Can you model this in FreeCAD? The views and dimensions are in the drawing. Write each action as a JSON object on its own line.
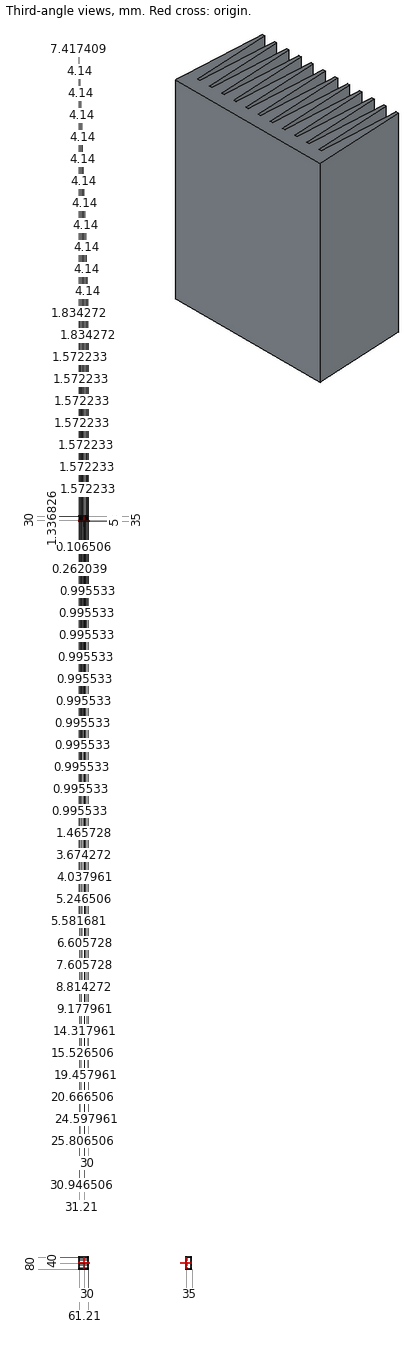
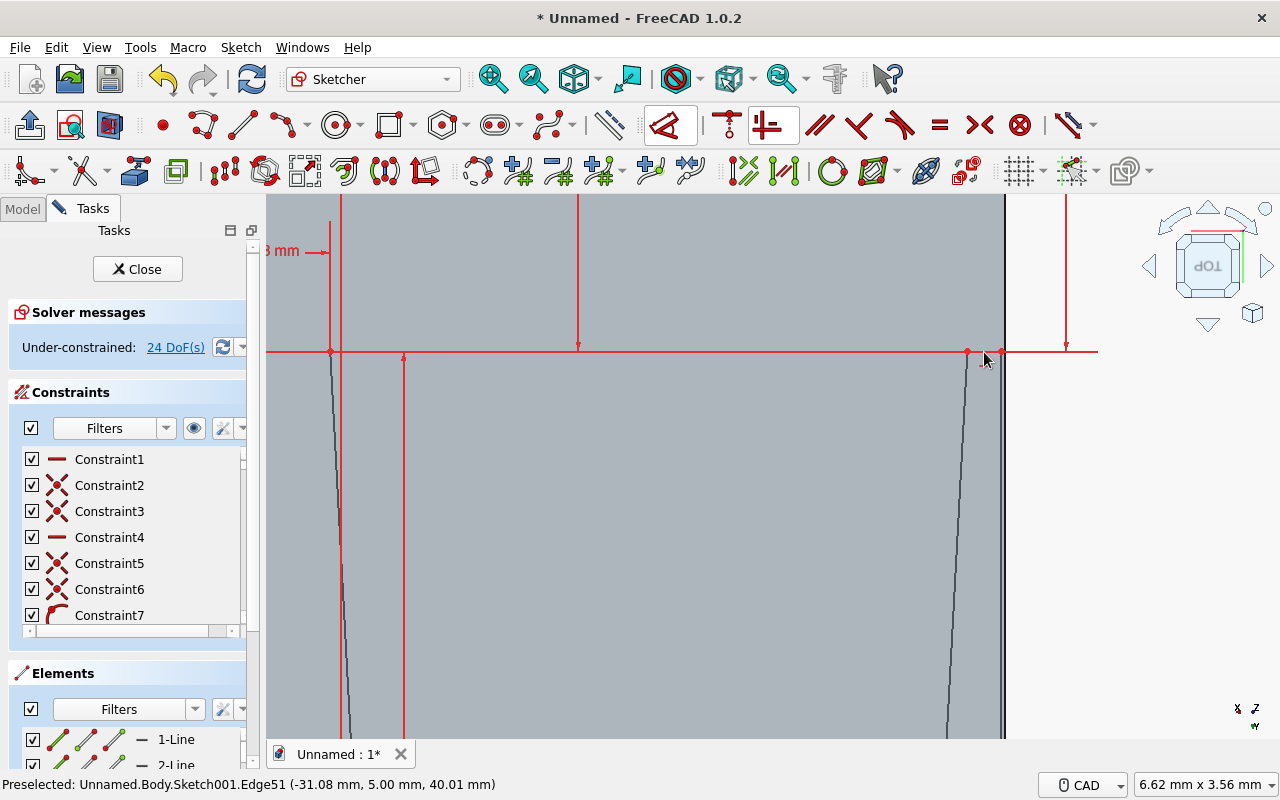
{"action": "left_click", "coordinate": [692, 126]}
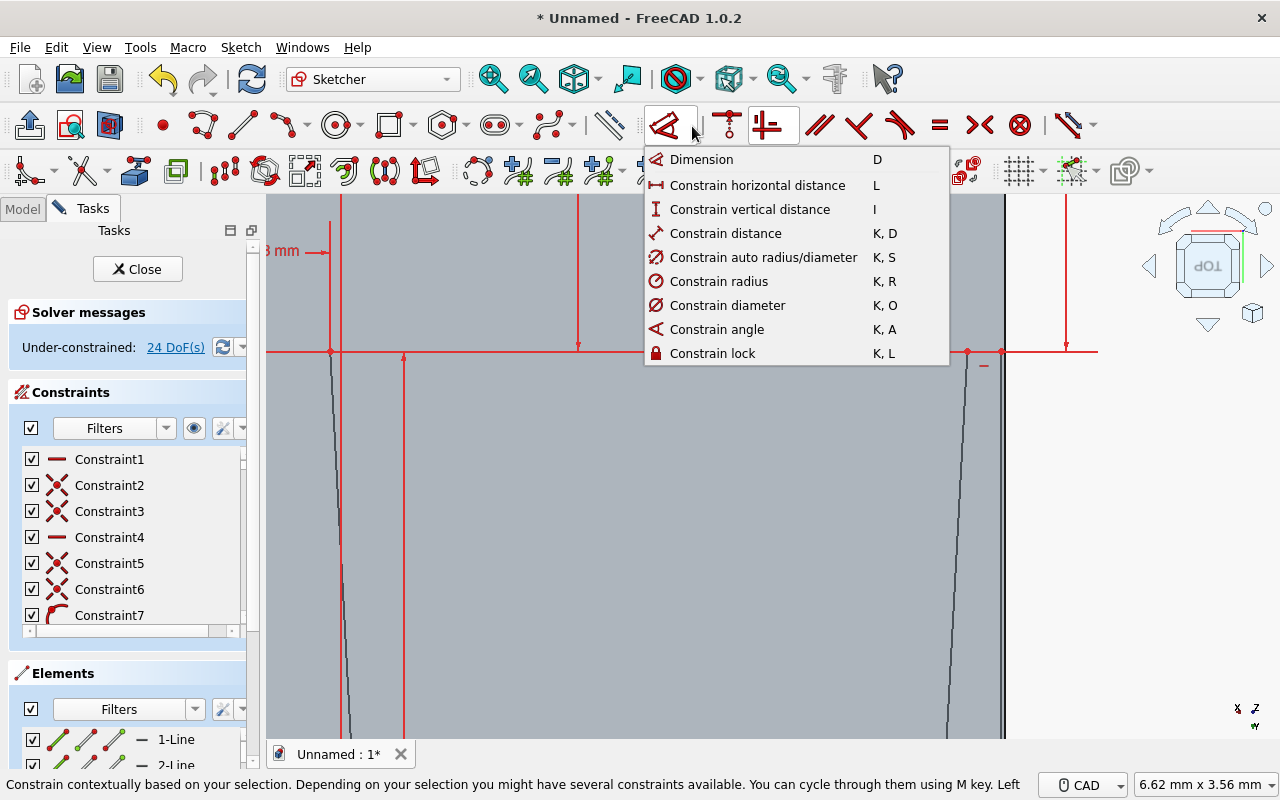
{"action": "left_click", "coordinate": [797, 185]}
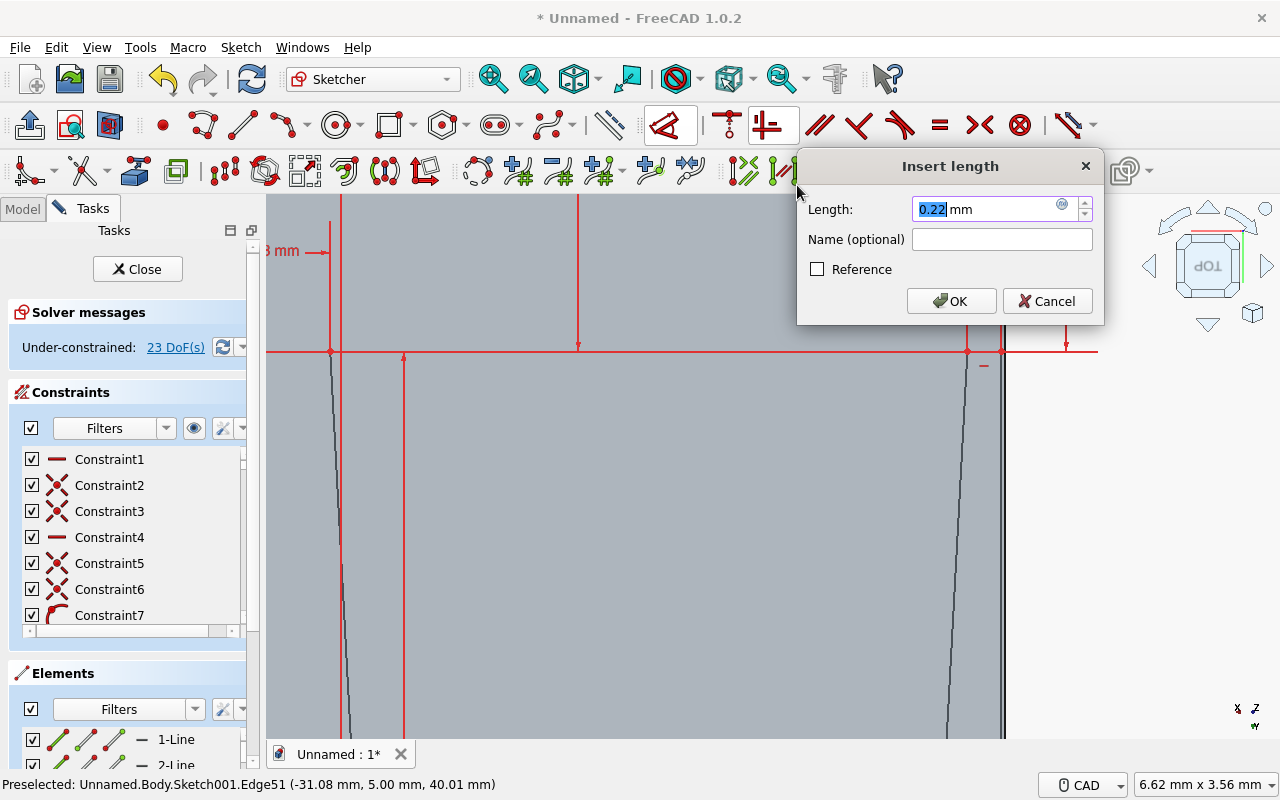
{"action": "type", "text": "0.262039"}
{"action": "key", "text": "Return"}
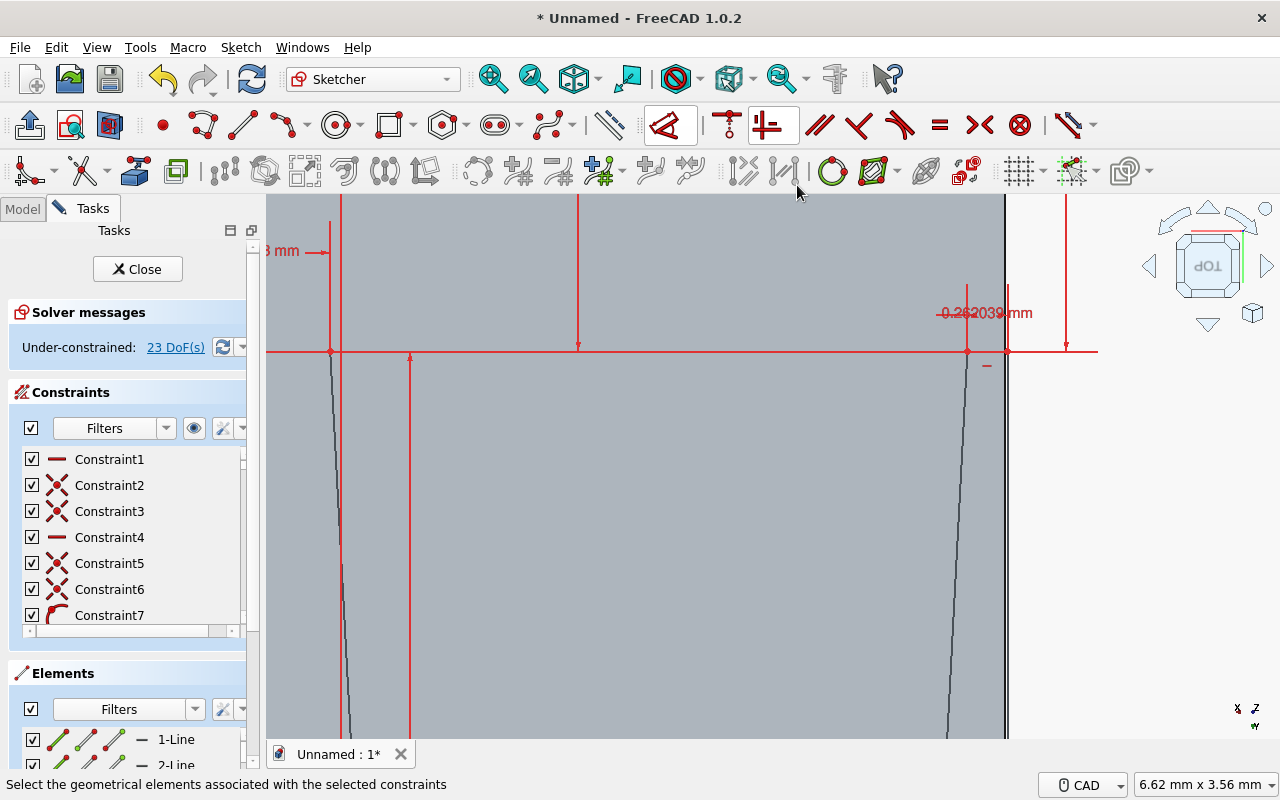
{"action": "scroll", "coordinate": [989, 350], "scroll_direction": "down", "scroll_amount": 14}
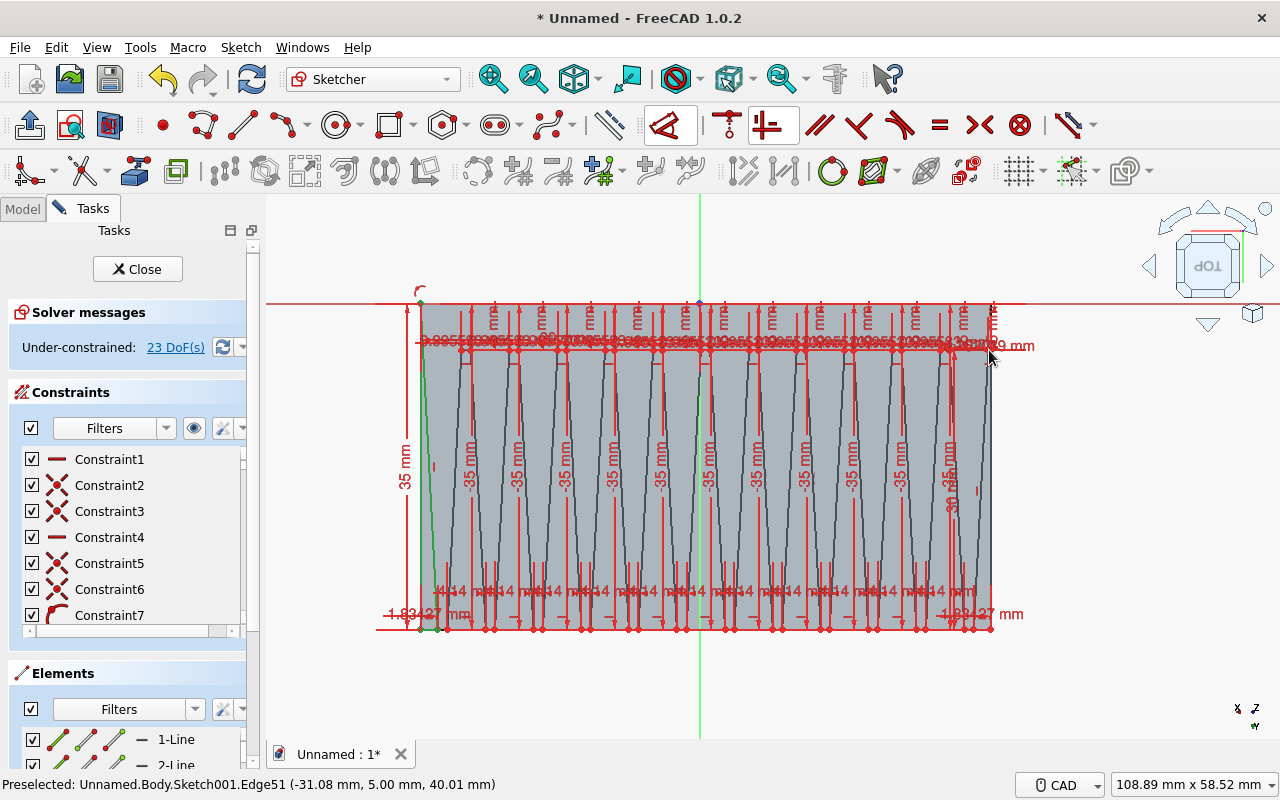
{"action": "scroll", "coordinate": [614, 350], "scroll_direction": "up", "scroll_amount": 2}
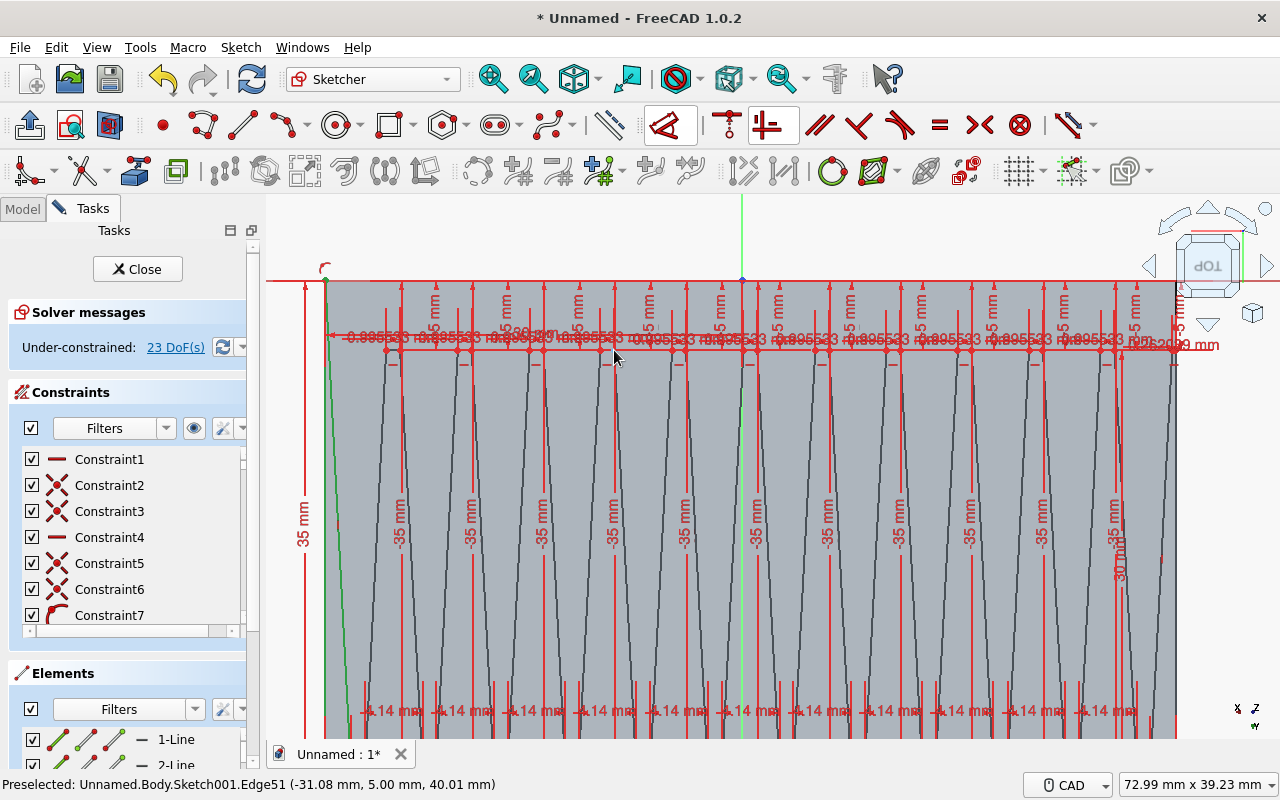
{"action": "left_click", "coordinate": [614, 350]}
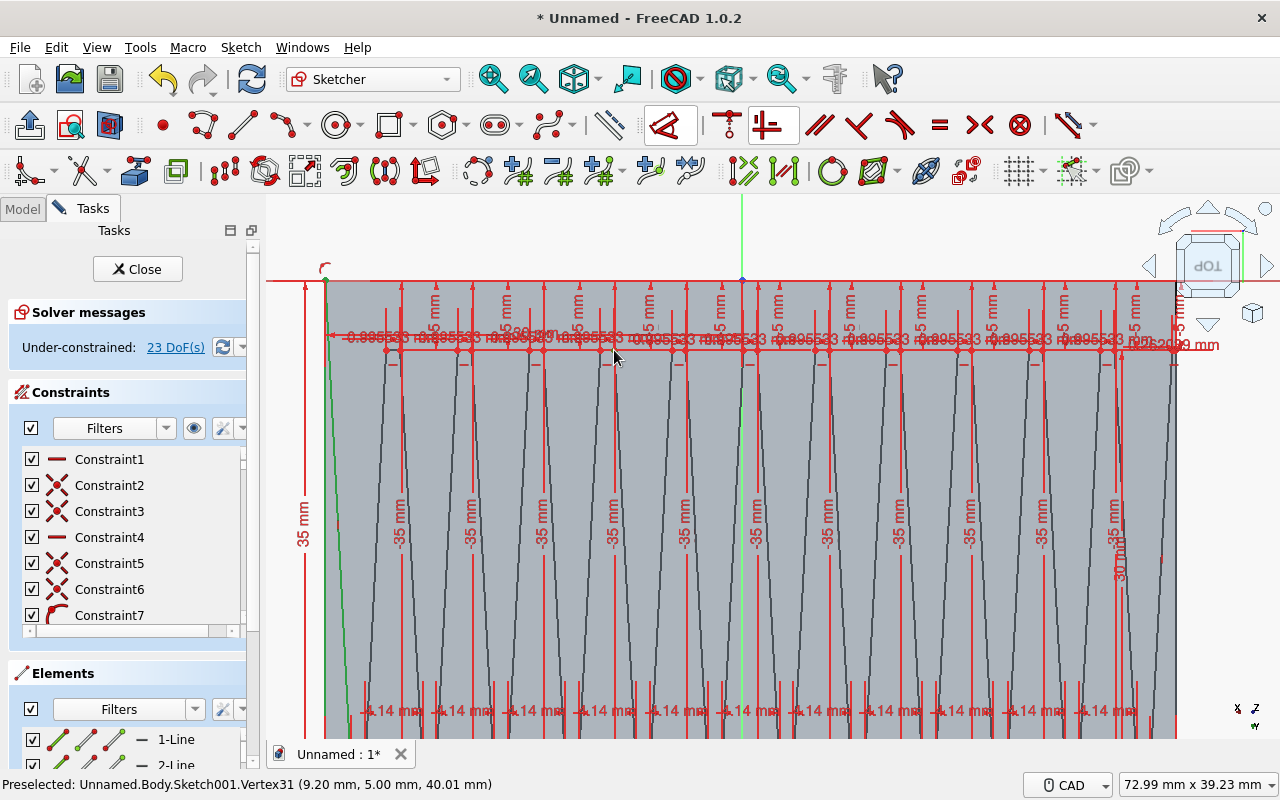
{"action": "left_click", "coordinate": [692, 126]}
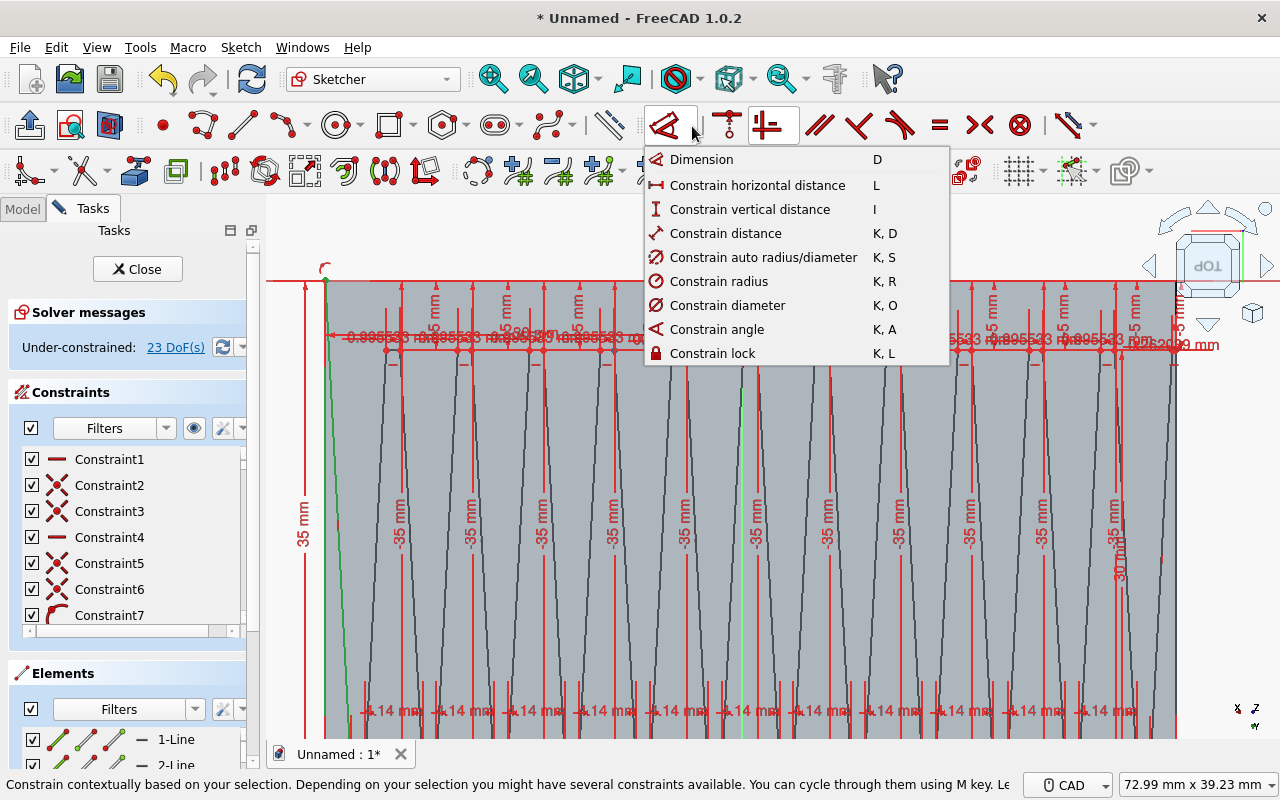
{"action": "left_click", "coordinate": [797, 185]}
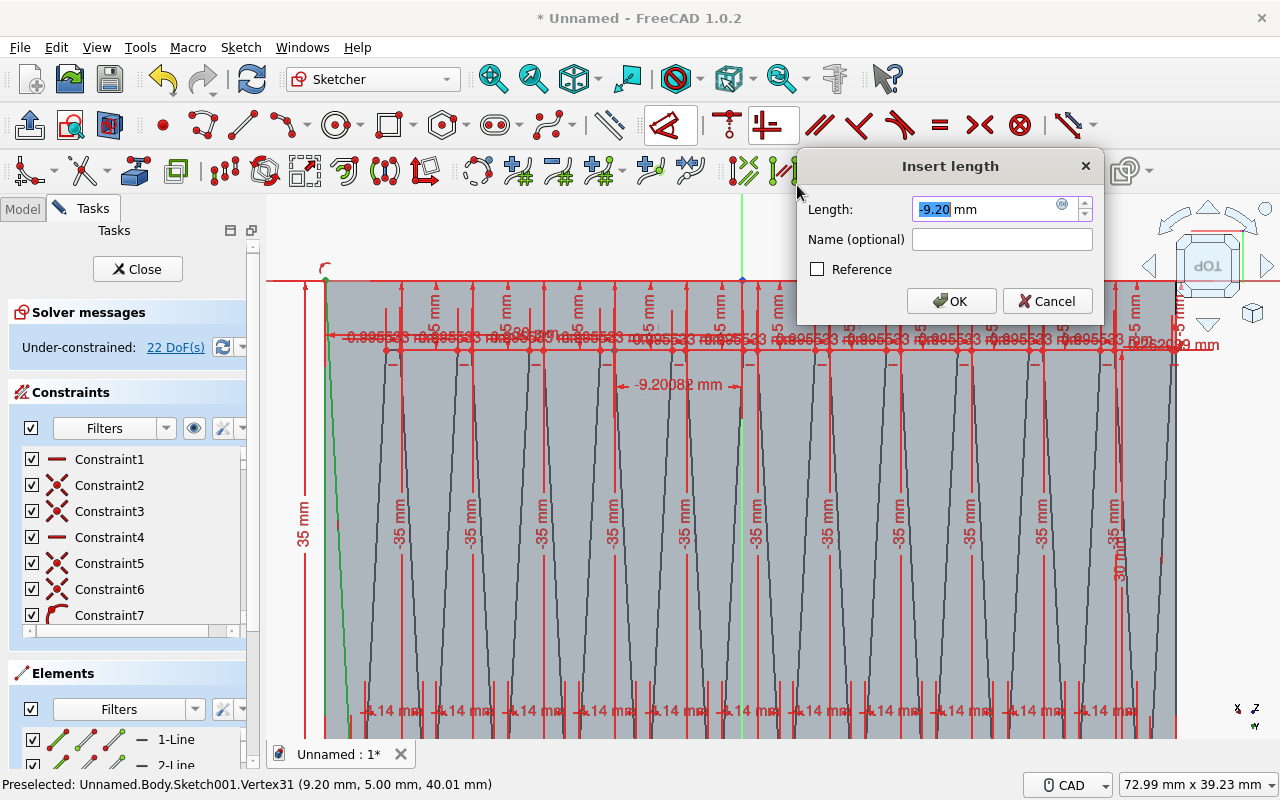
{"action": "type", "text": "-9.177961"}
{"action": "key", "text": "Return"}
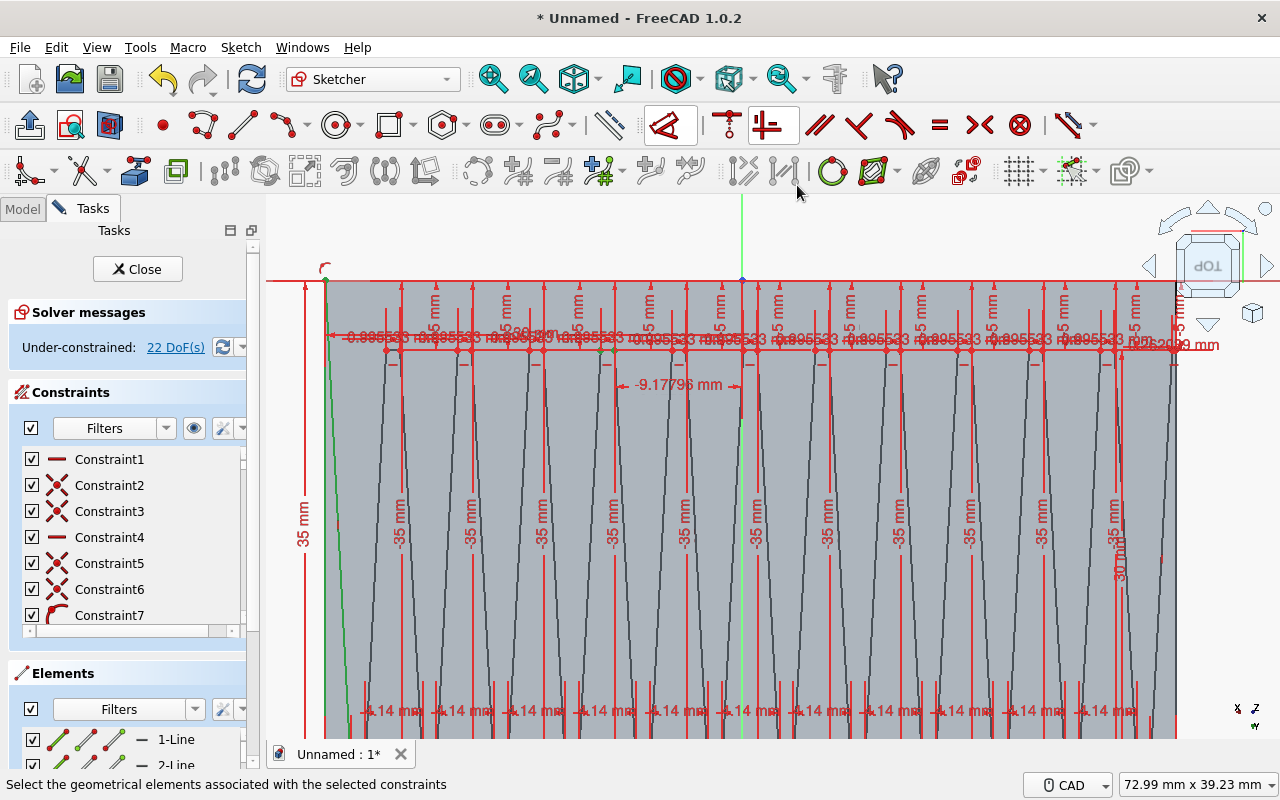
{"action": "scroll", "coordinate": [611, 349], "scroll_direction": "down", "scroll_amount": 2}